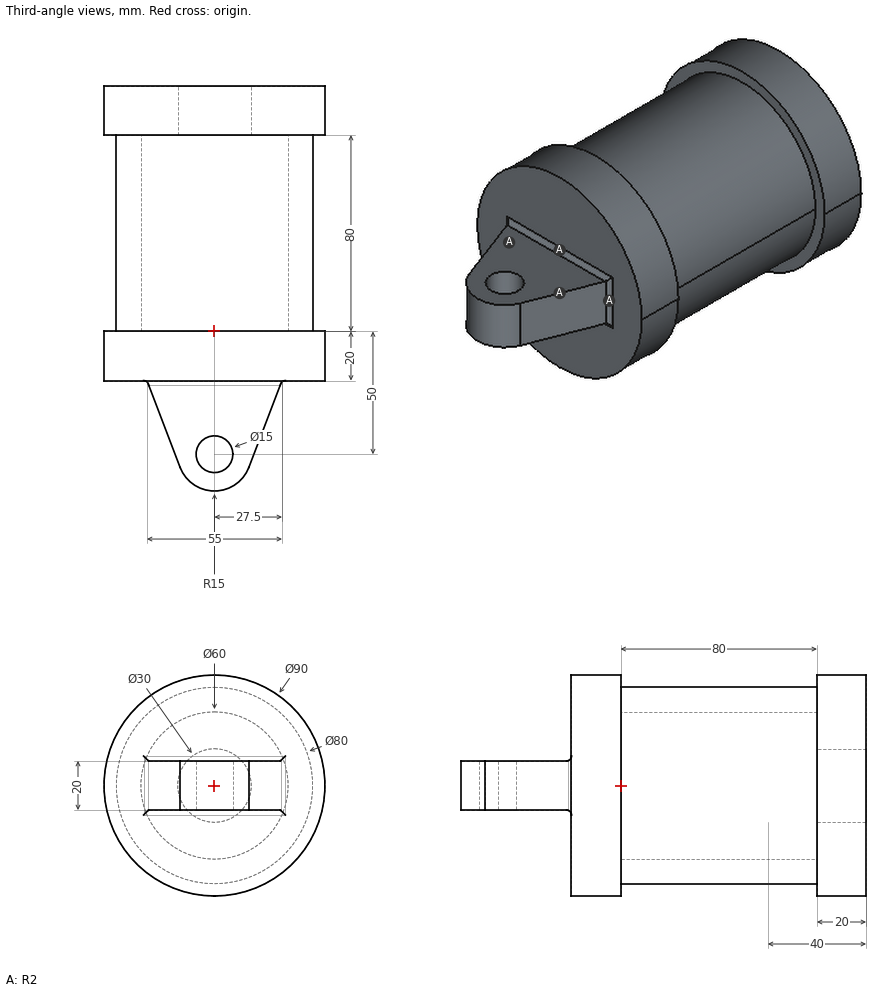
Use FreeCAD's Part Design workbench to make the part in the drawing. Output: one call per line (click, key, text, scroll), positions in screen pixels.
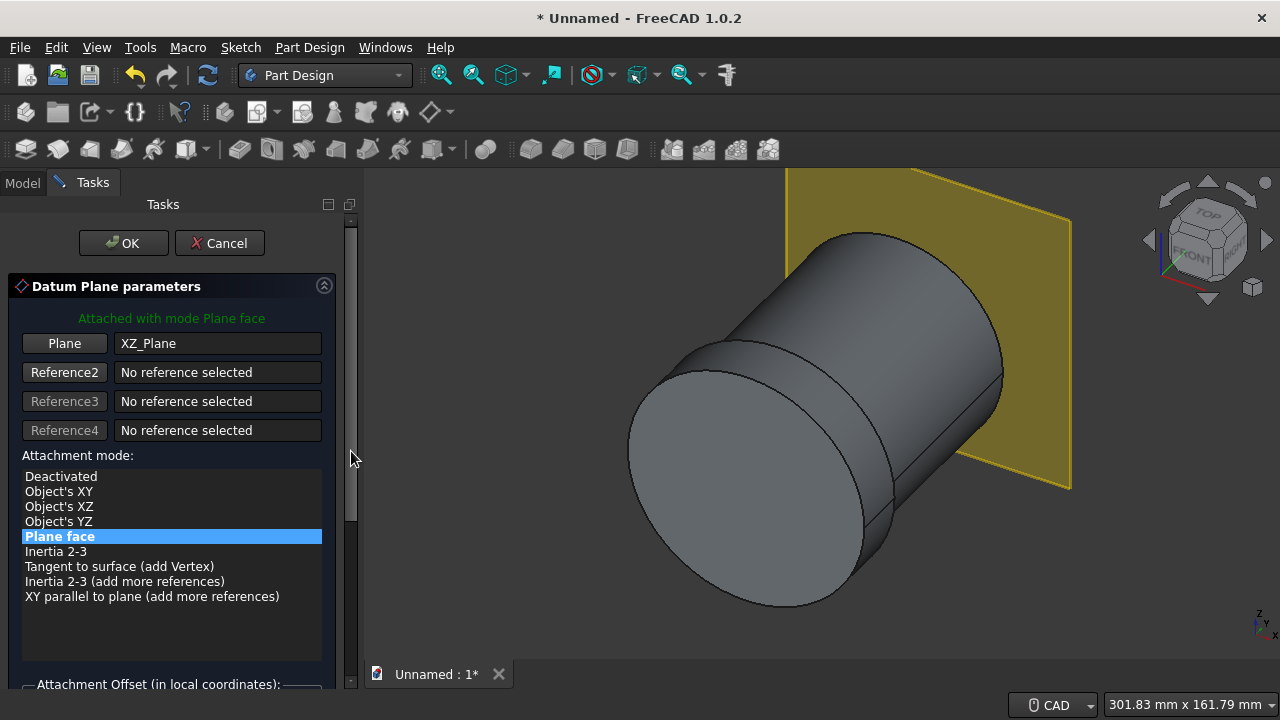
click(124, 243)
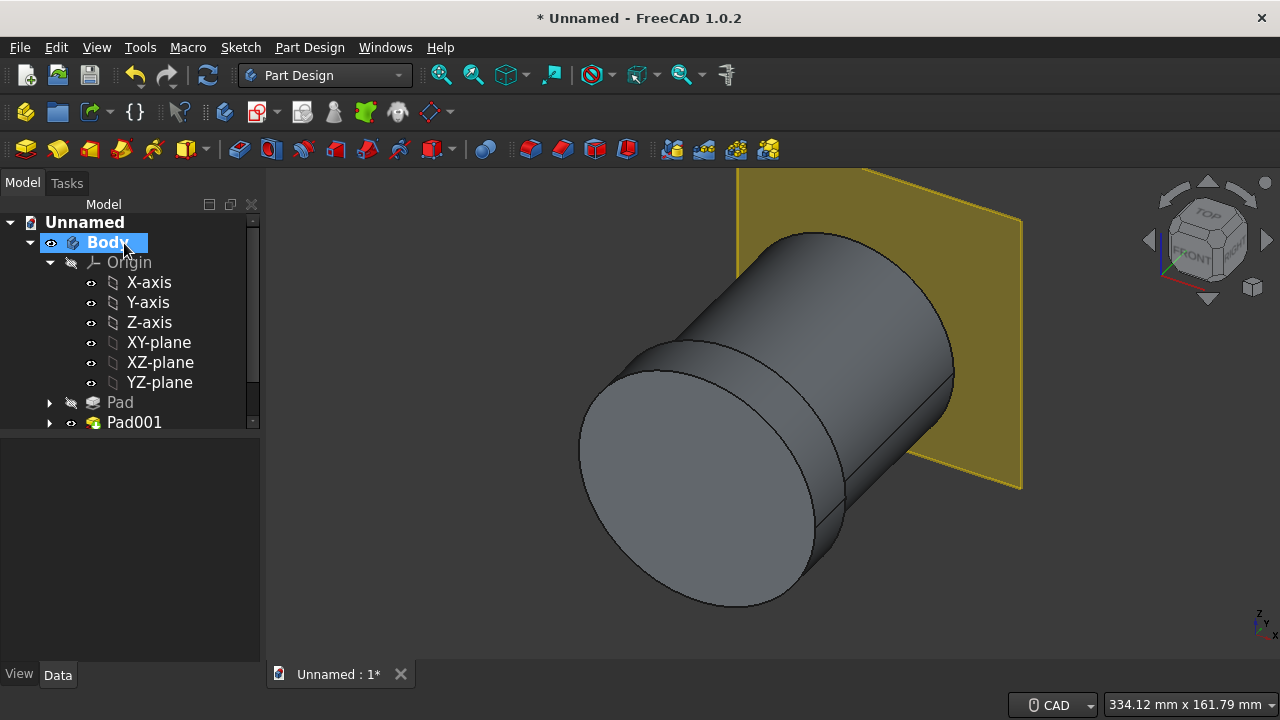
scroll(100, 318, down, 3)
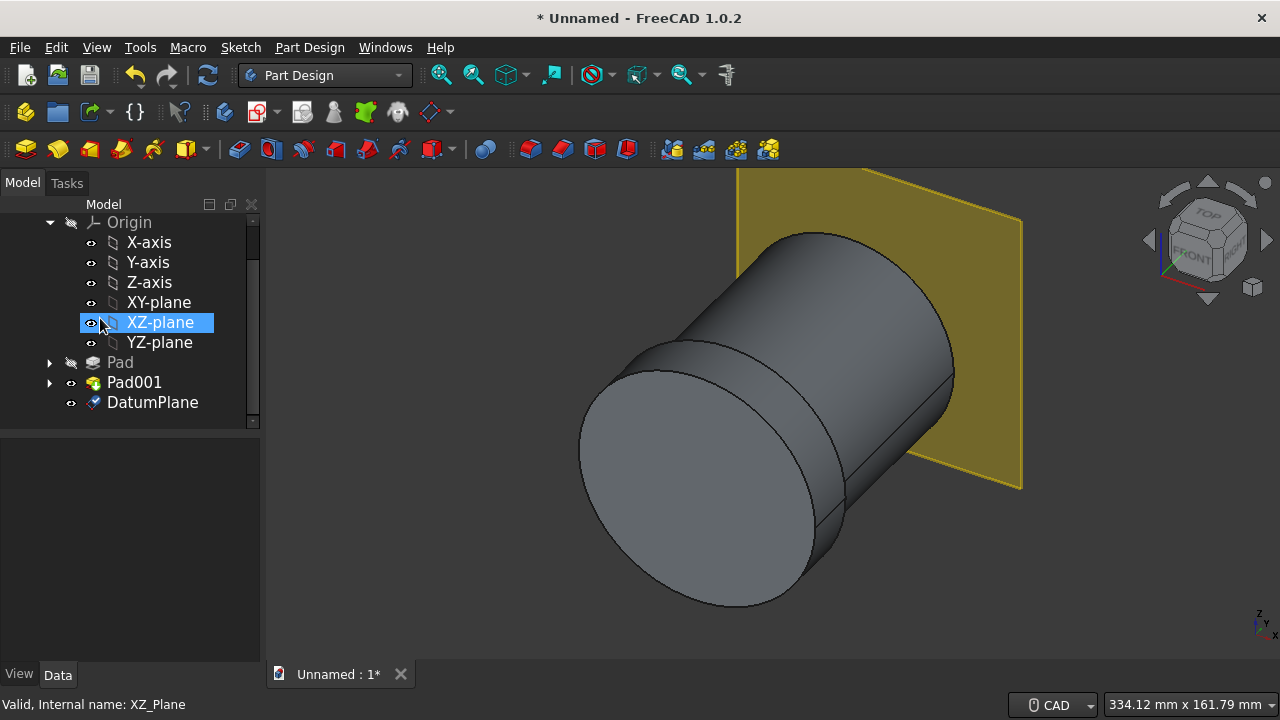
click(116, 403)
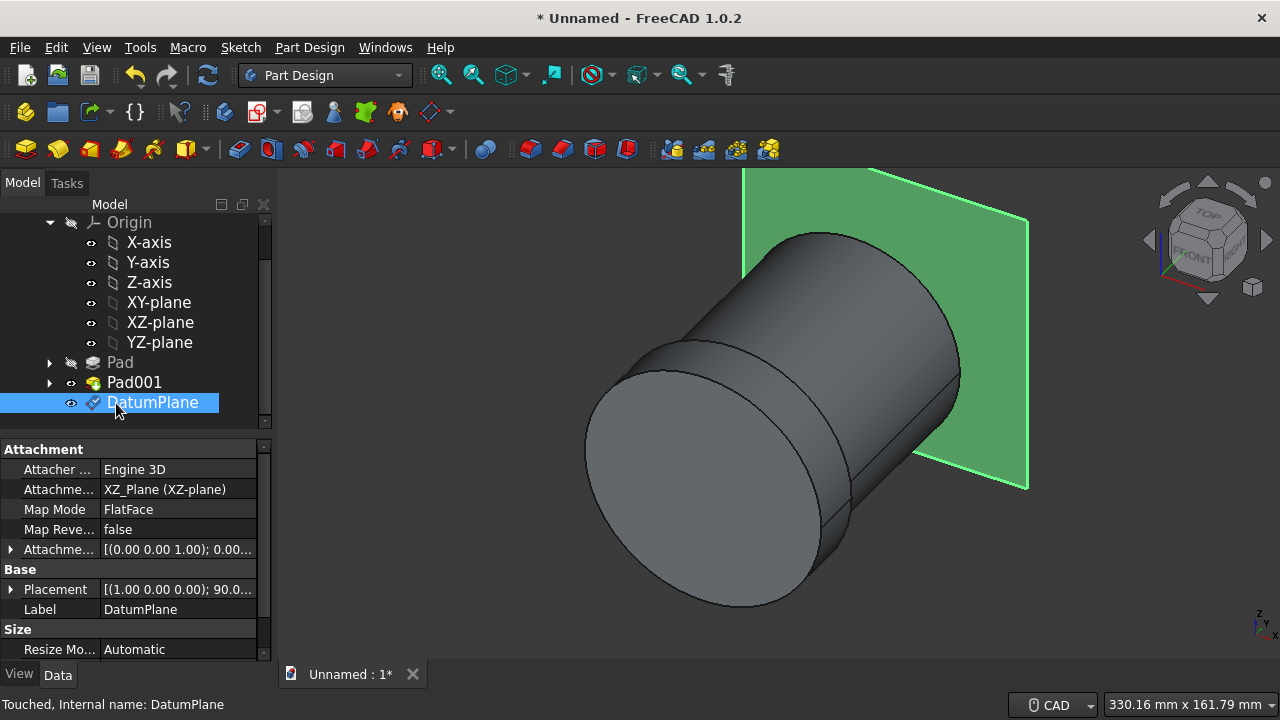
click(258, 112)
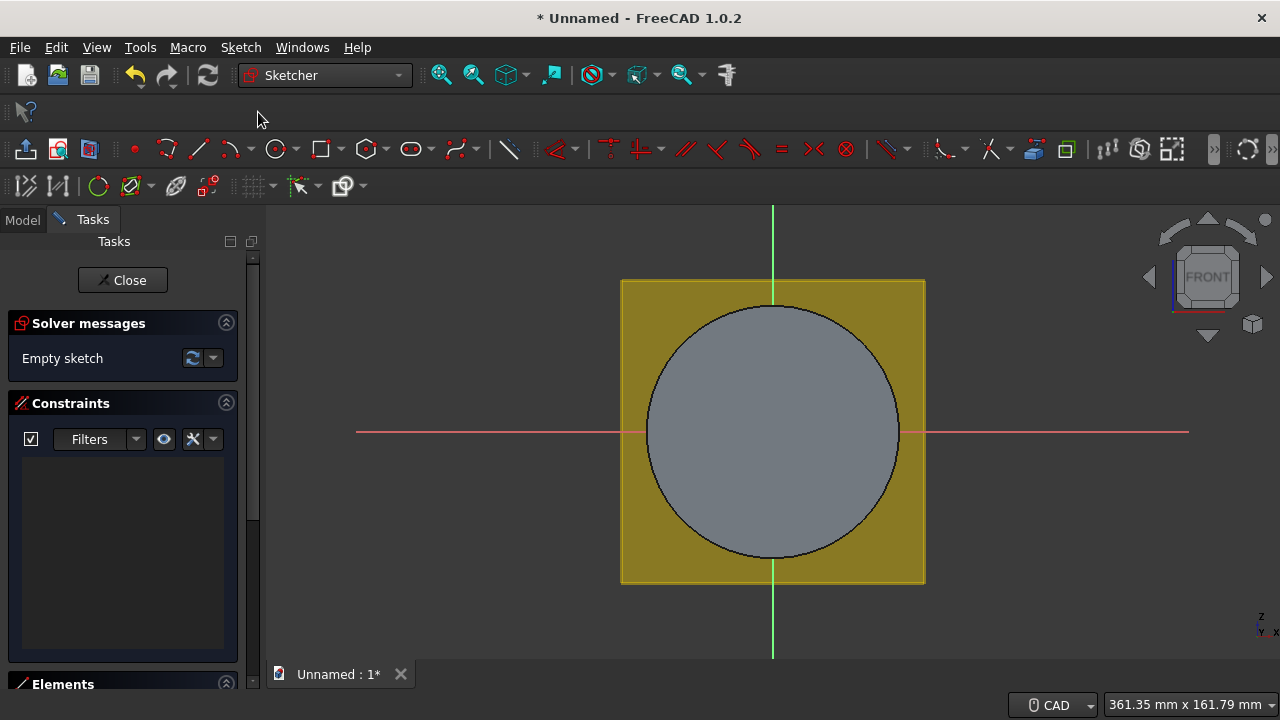
click(90, 150)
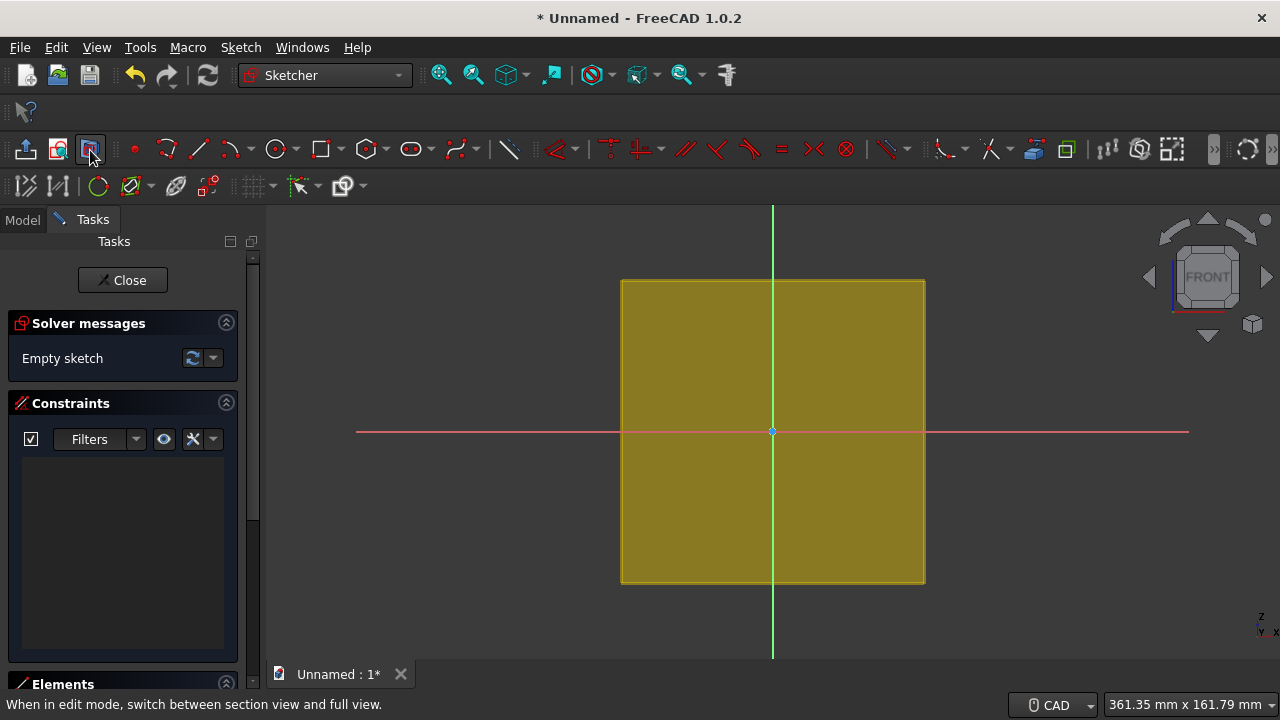
key(g)
key(c)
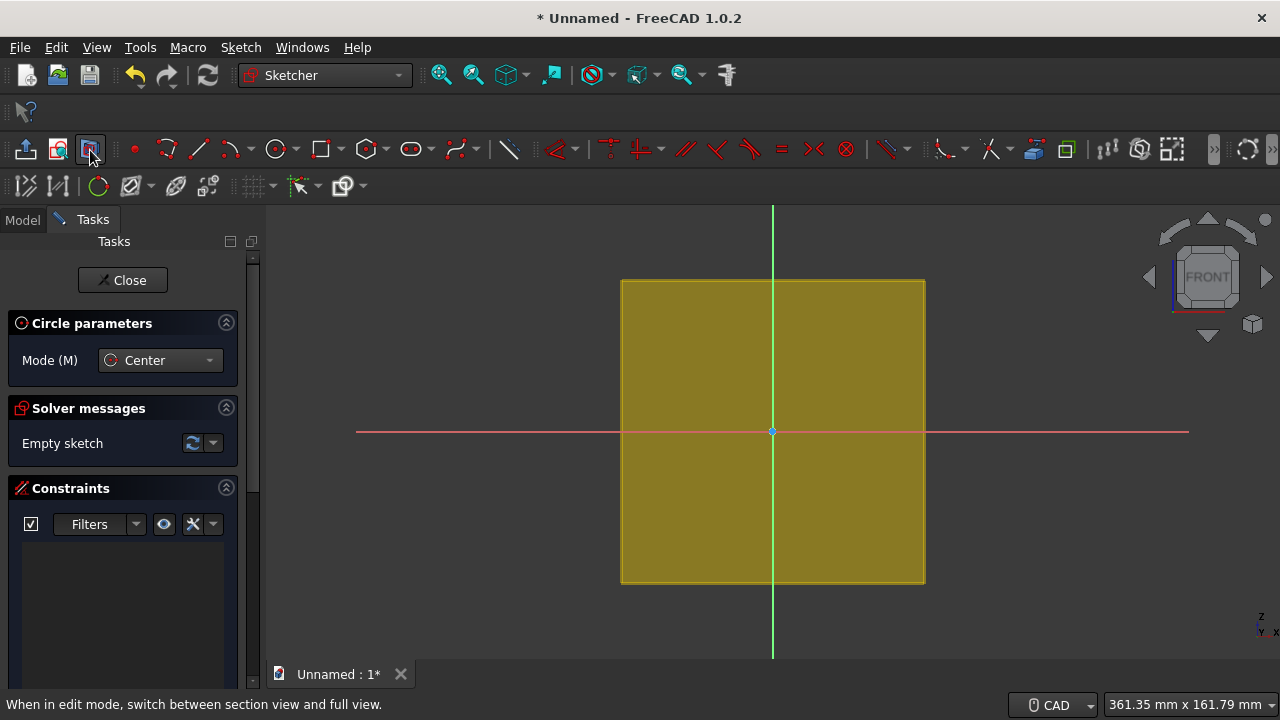
click(773, 432)
move(862, 343)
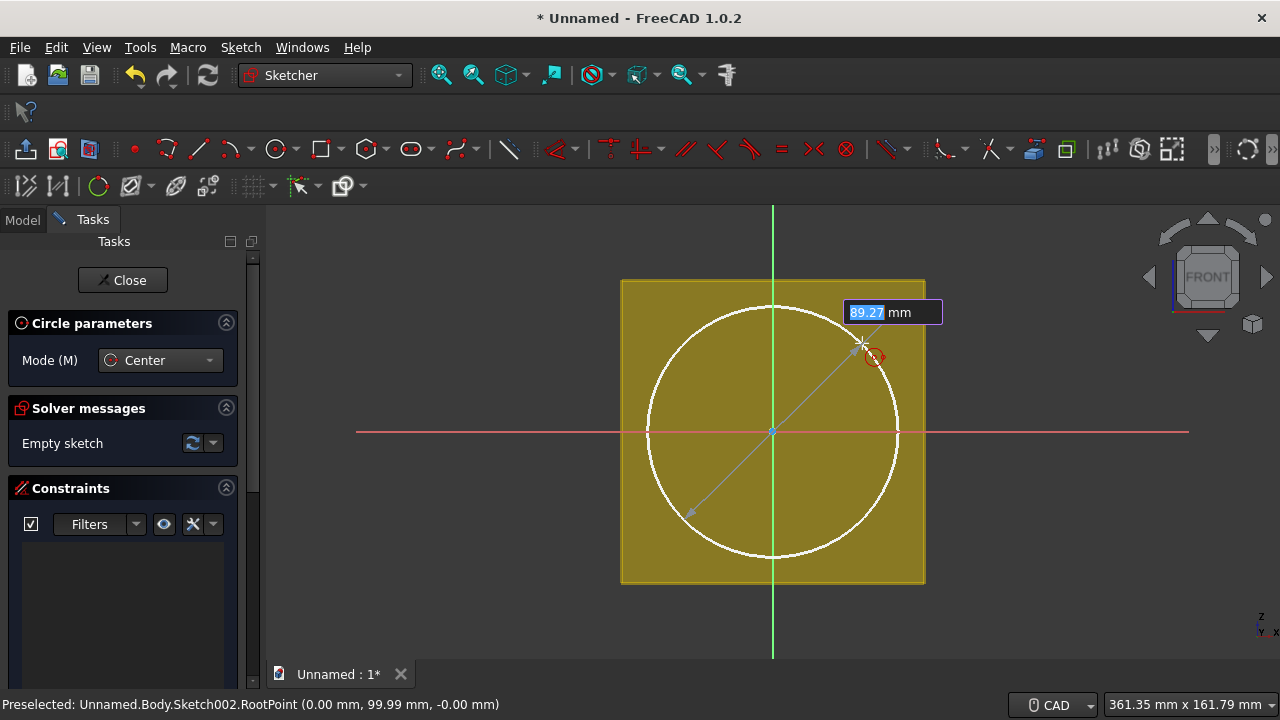
text(90)
key(Return)
key(Escape)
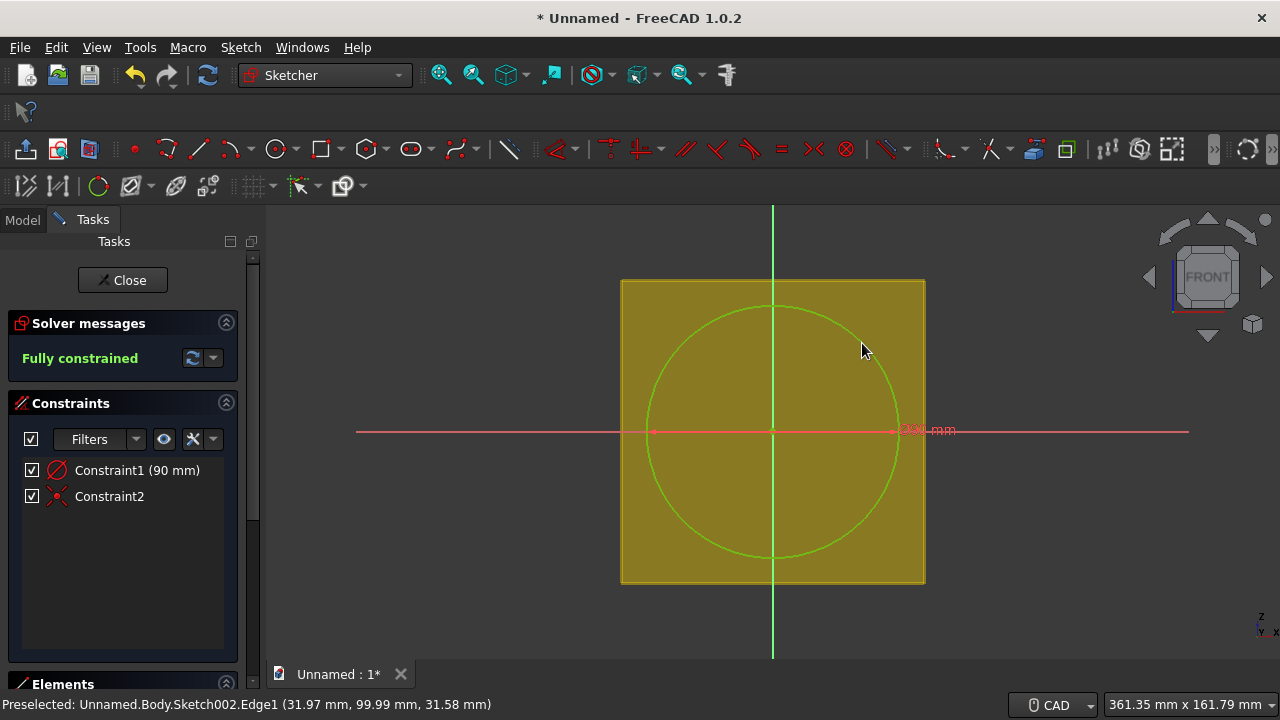
click(123, 280)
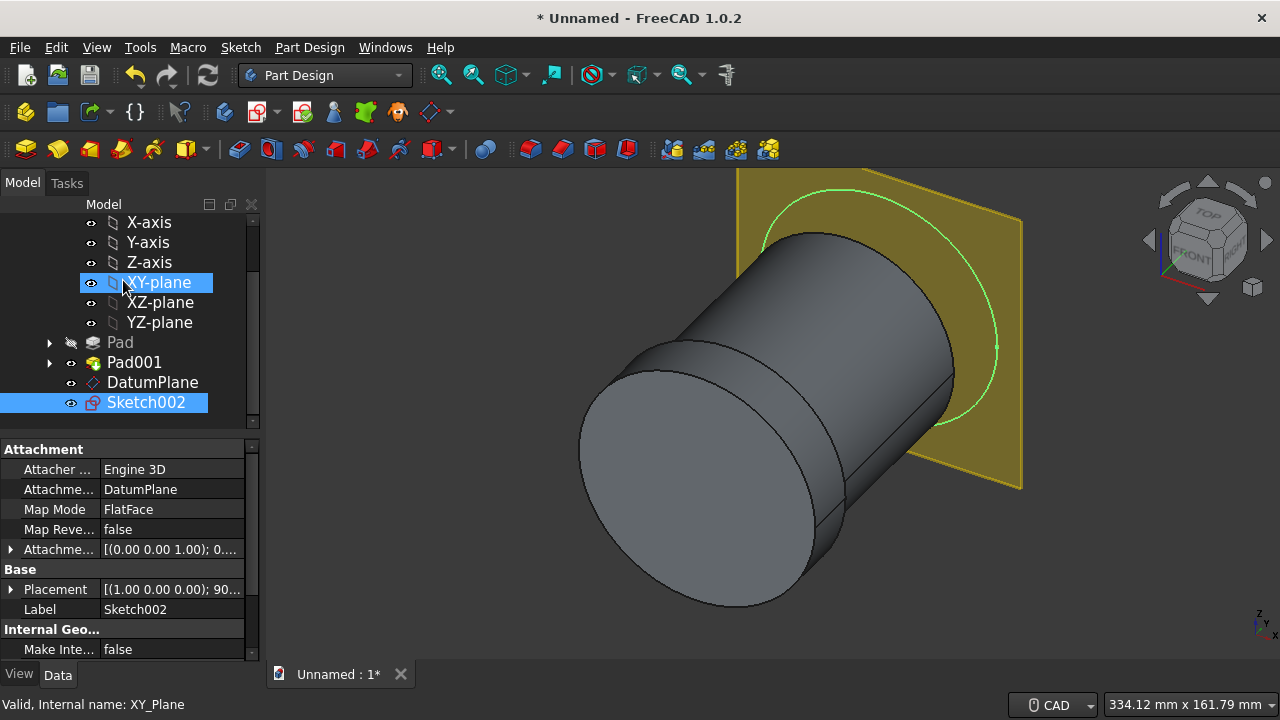
click(26, 150)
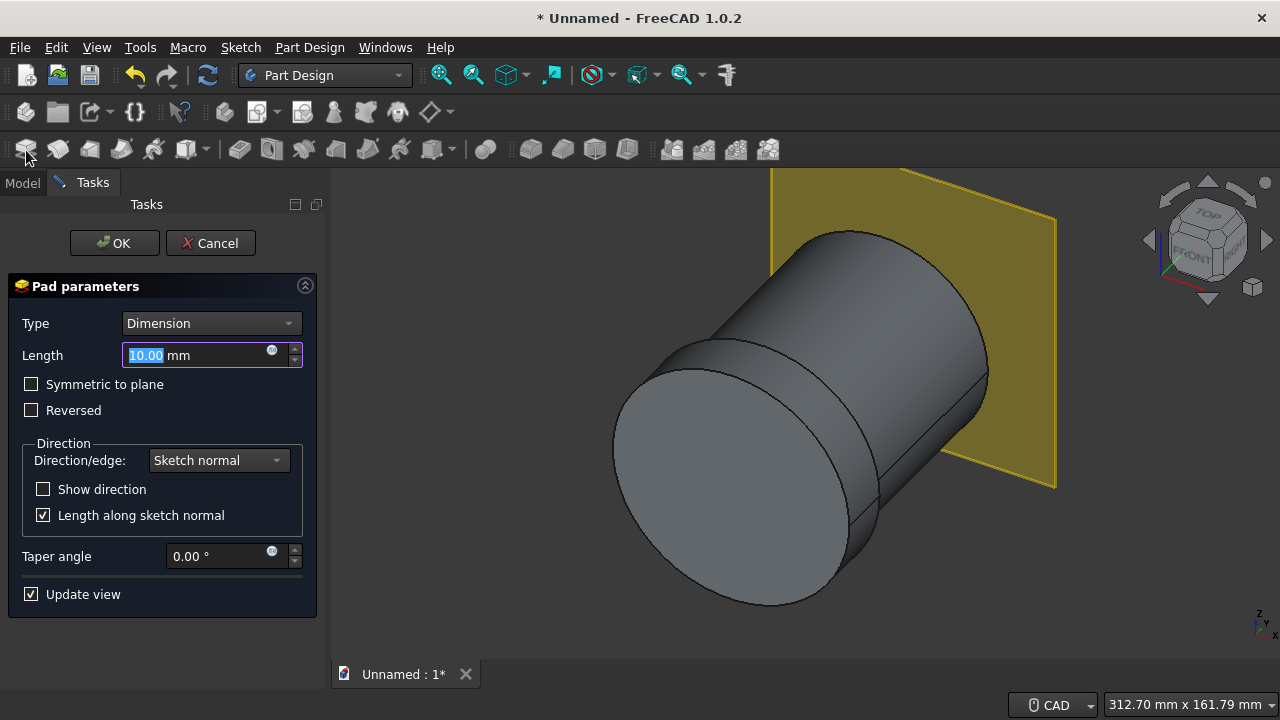
text(20)
key(Tab)